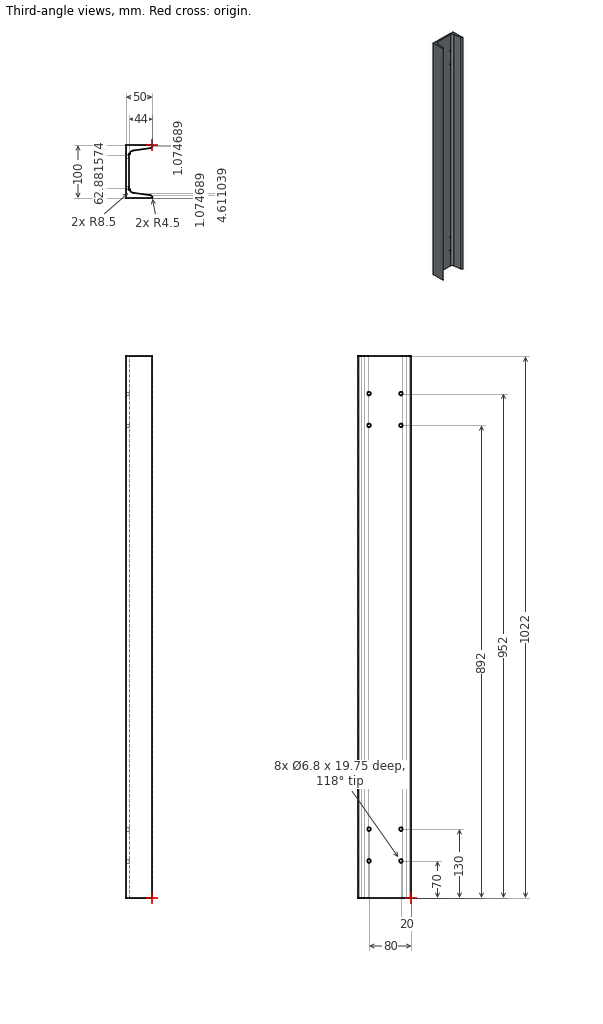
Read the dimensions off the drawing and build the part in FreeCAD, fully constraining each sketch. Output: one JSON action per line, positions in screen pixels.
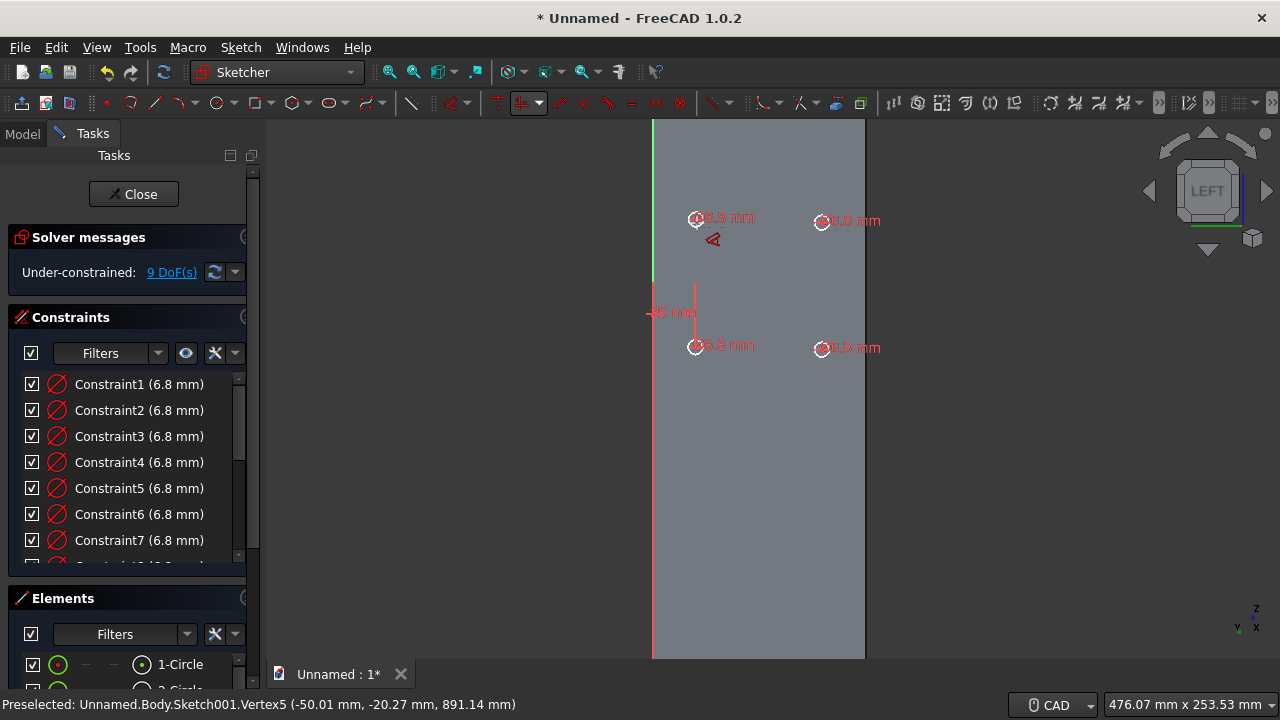
{"action": "left_click", "coordinate": [696, 220]}
{"action": "left_click", "coordinate": [674, 186]}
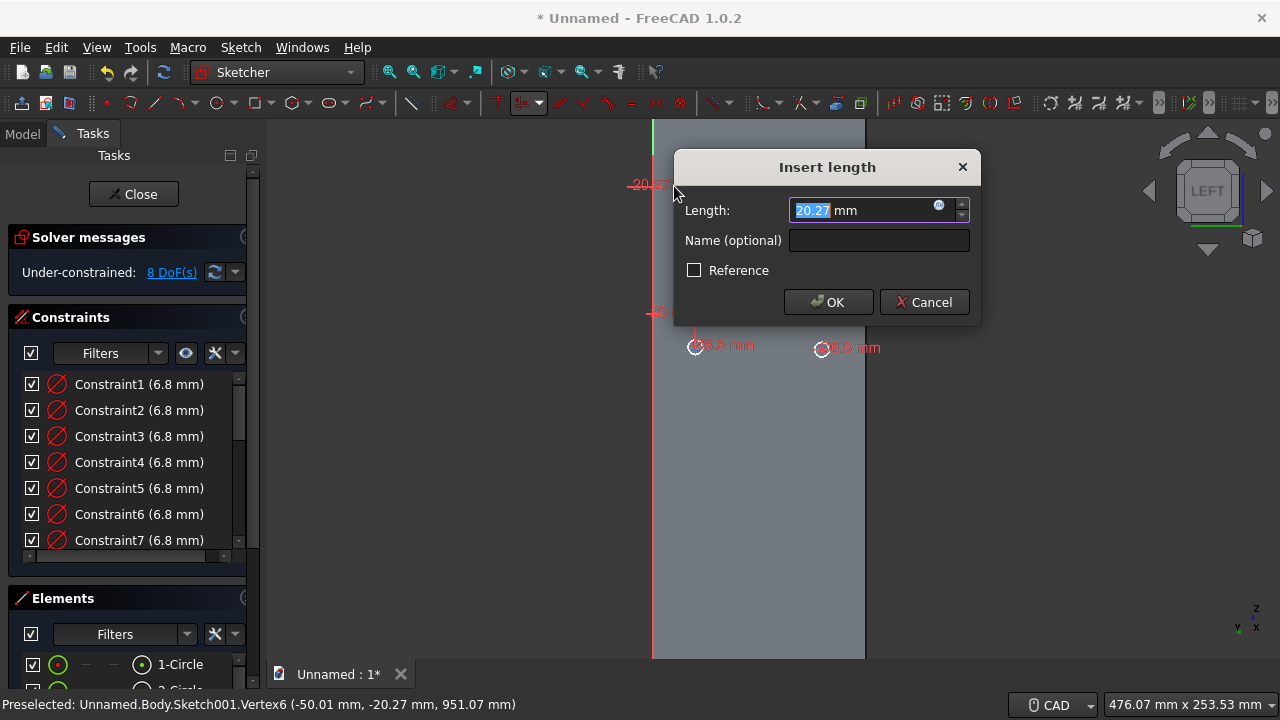
{"action": "type", "text": "20"}
{"action": "key", "text": "Return"}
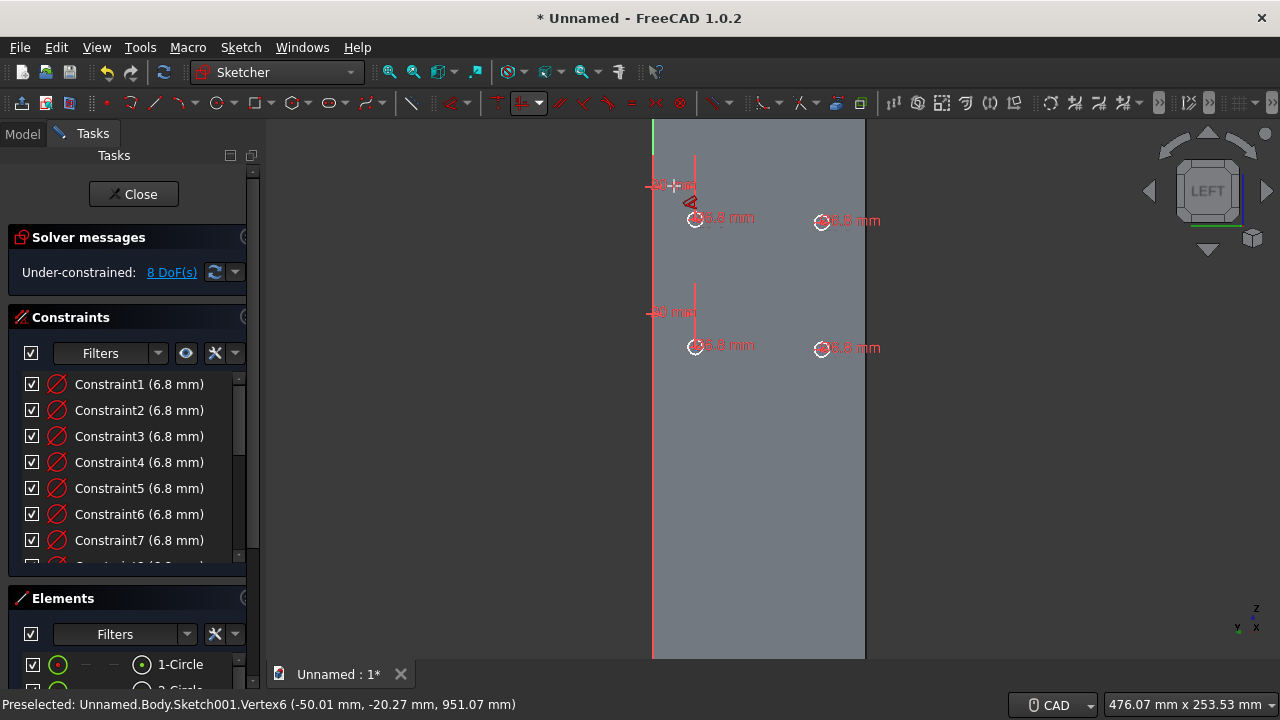
{"action": "scroll", "coordinate": [697, 223], "scroll_direction": "down", "scroll_amount": 9}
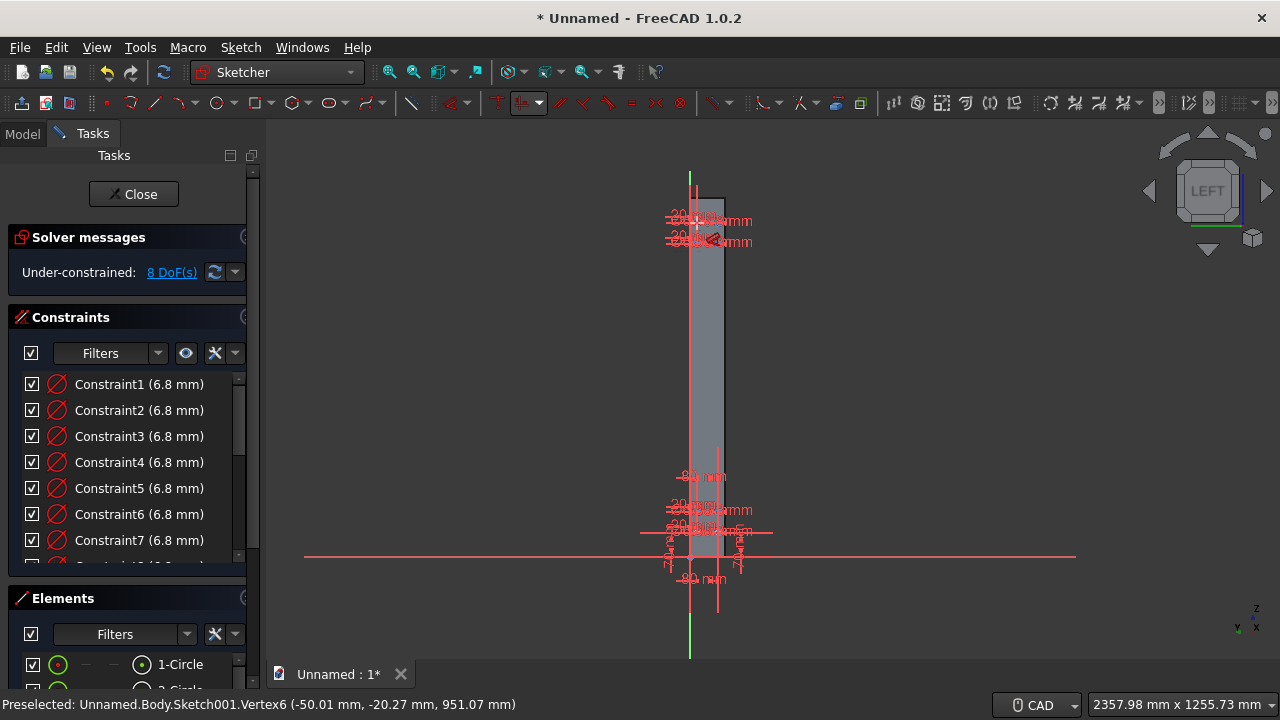
{"action": "scroll", "coordinate": [718, 223], "scroll_direction": "up", "scroll_amount": 2}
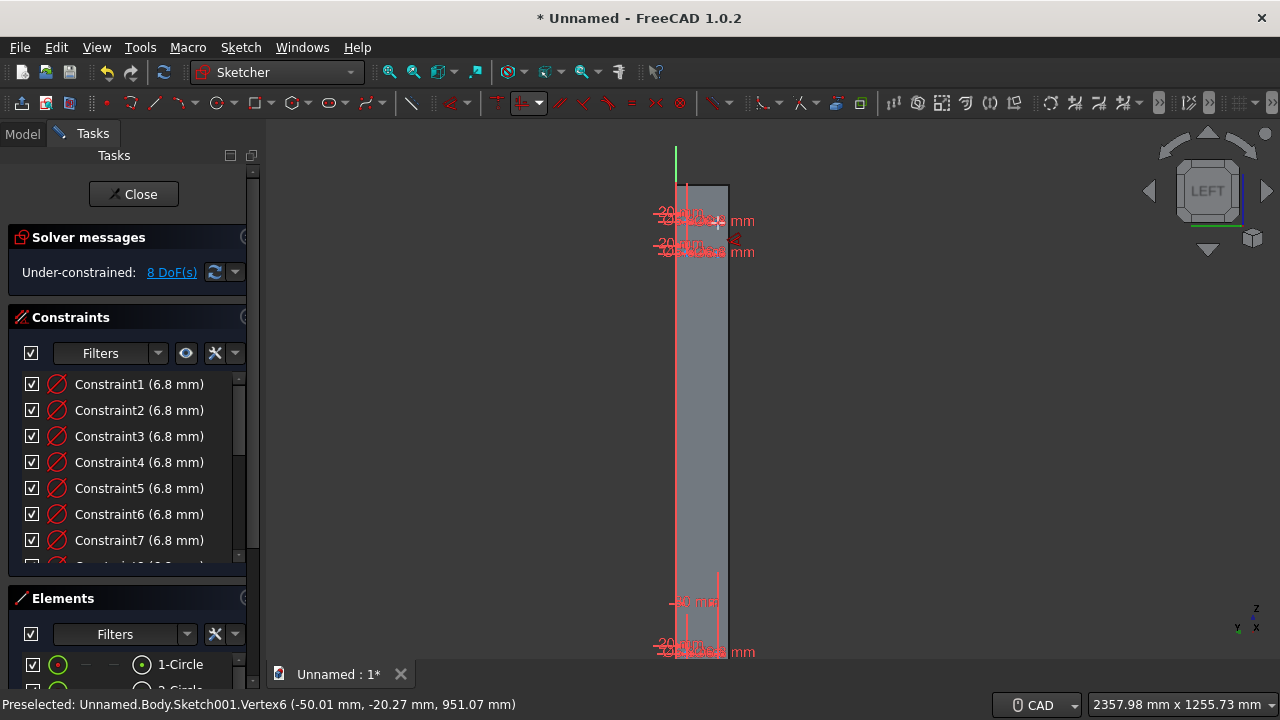
{"action": "left_click", "coordinate": [718, 223]}
{"action": "left_click", "coordinate": [697, 189]}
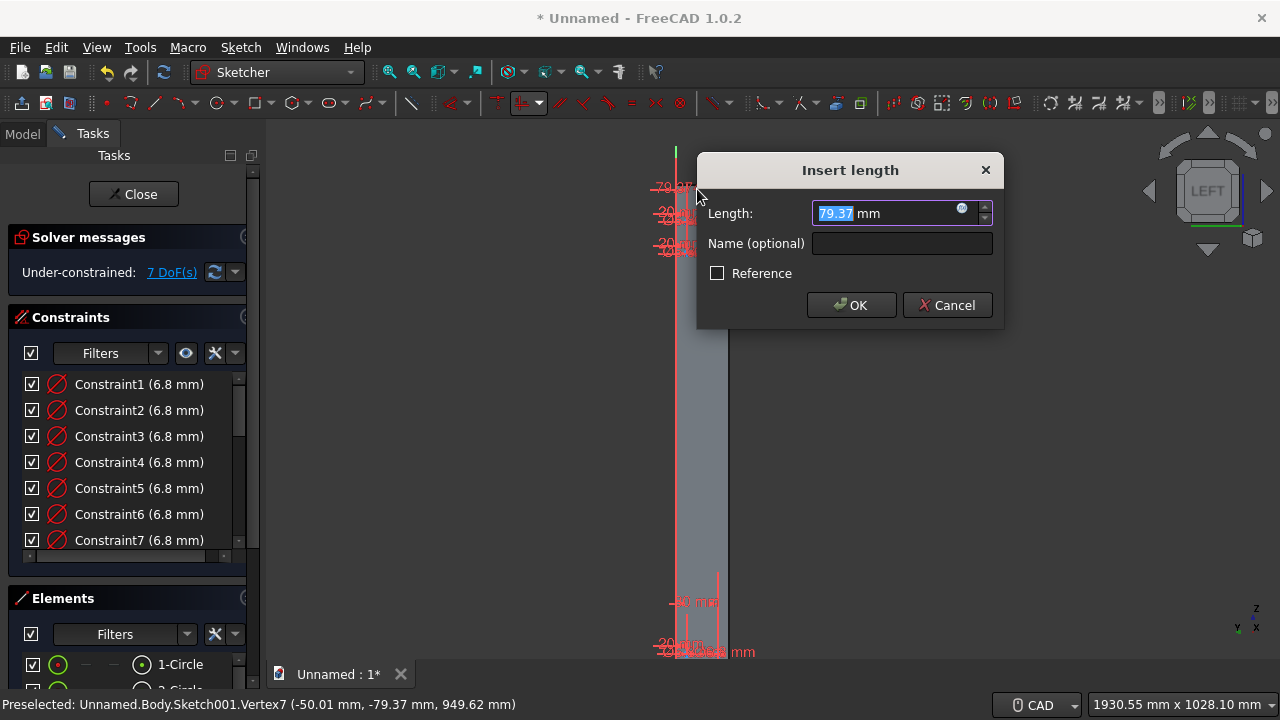
{"action": "type", "text": "80"}
{"action": "key", "text": "Return"}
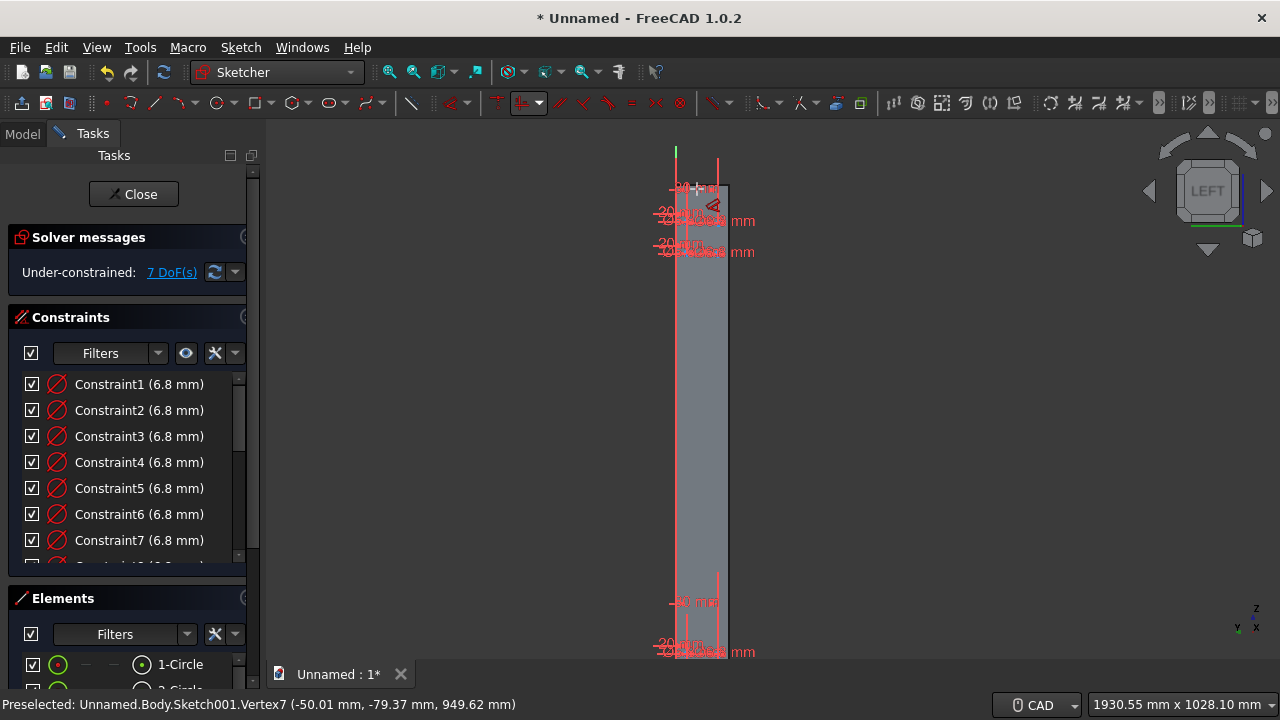
{"action": "left_click", "coordinate": [718, 254]}
{"action": "left_click", "coordinate": [697, 148]}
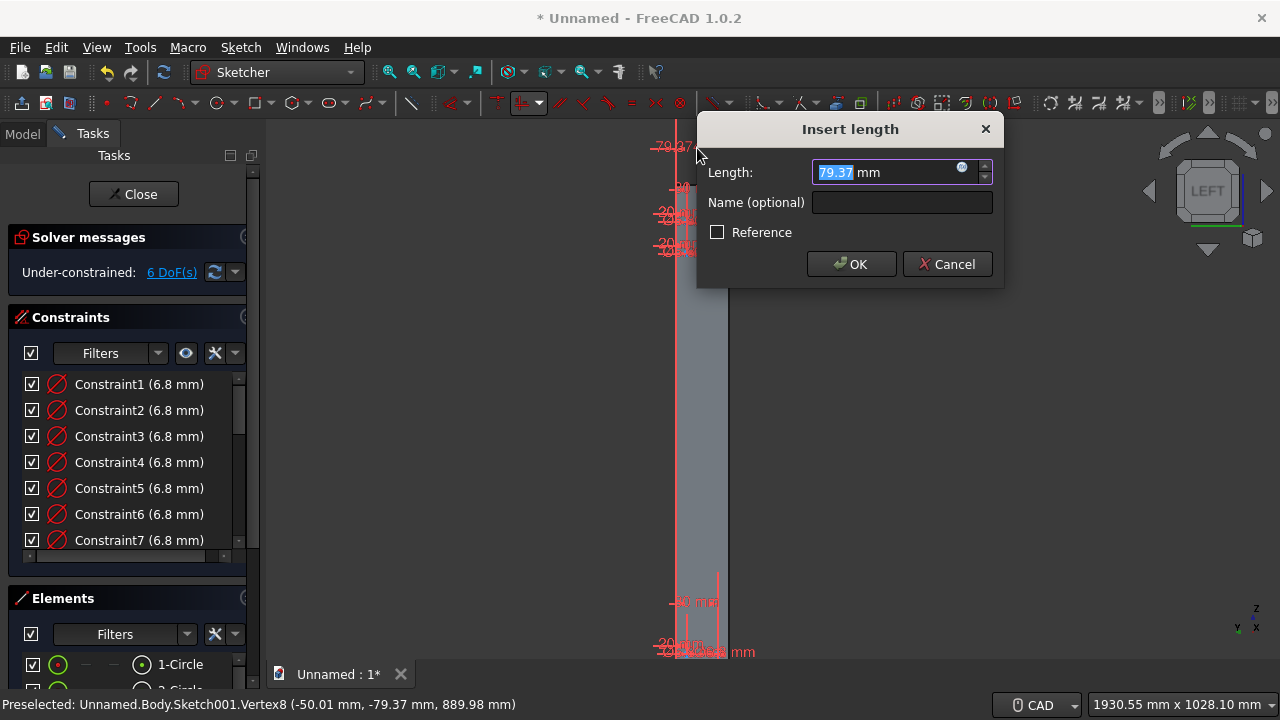
{"action": "type", "text": "80"}
{"action": "key", "text": "Return"}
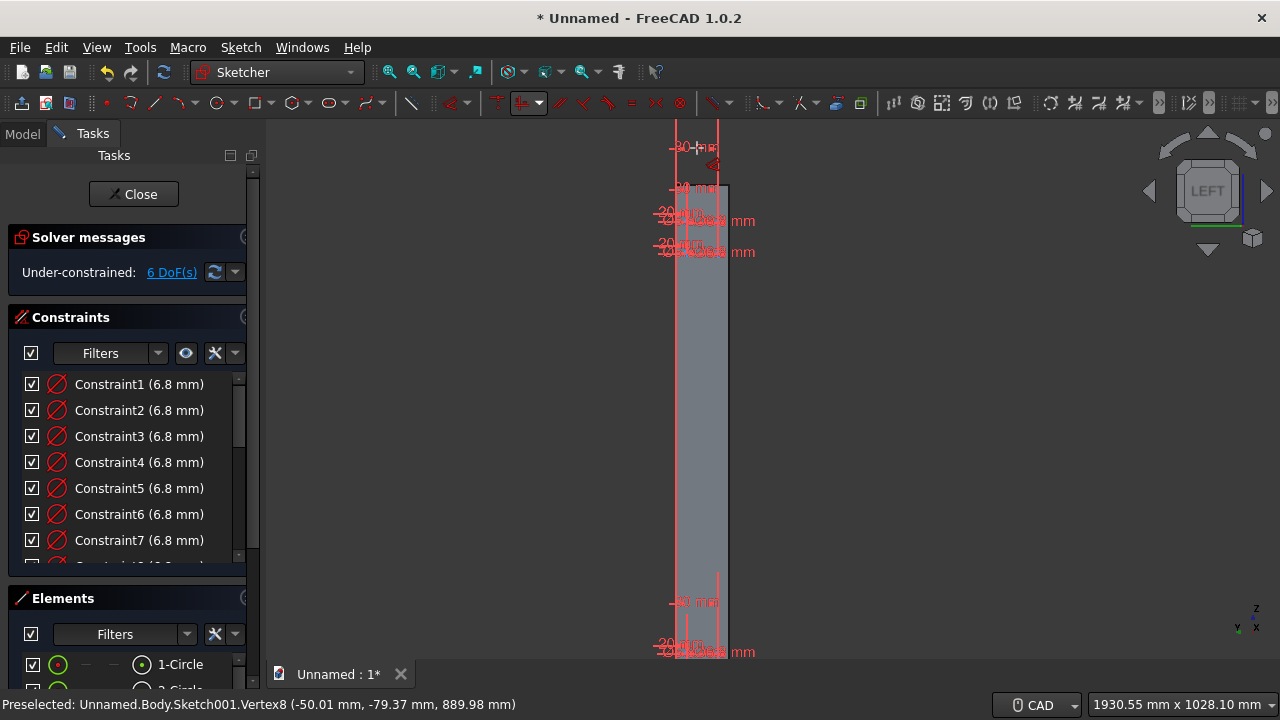
{"action": "scroll", "coordinate": [718, 222], "scroll_direction": "down", "scroll_amount": 2}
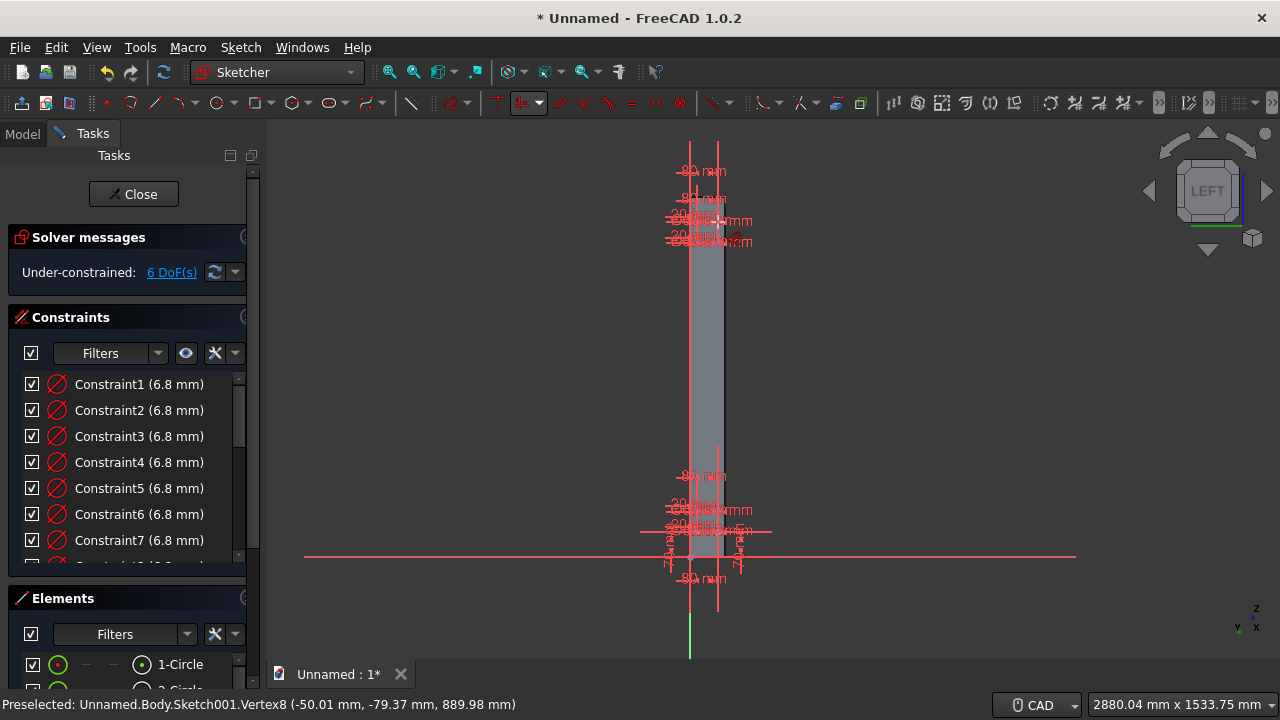
{"action": "left_click", "coordinate": [697, 512]}
{"action": "left_click", "coordinate": [608, 524]}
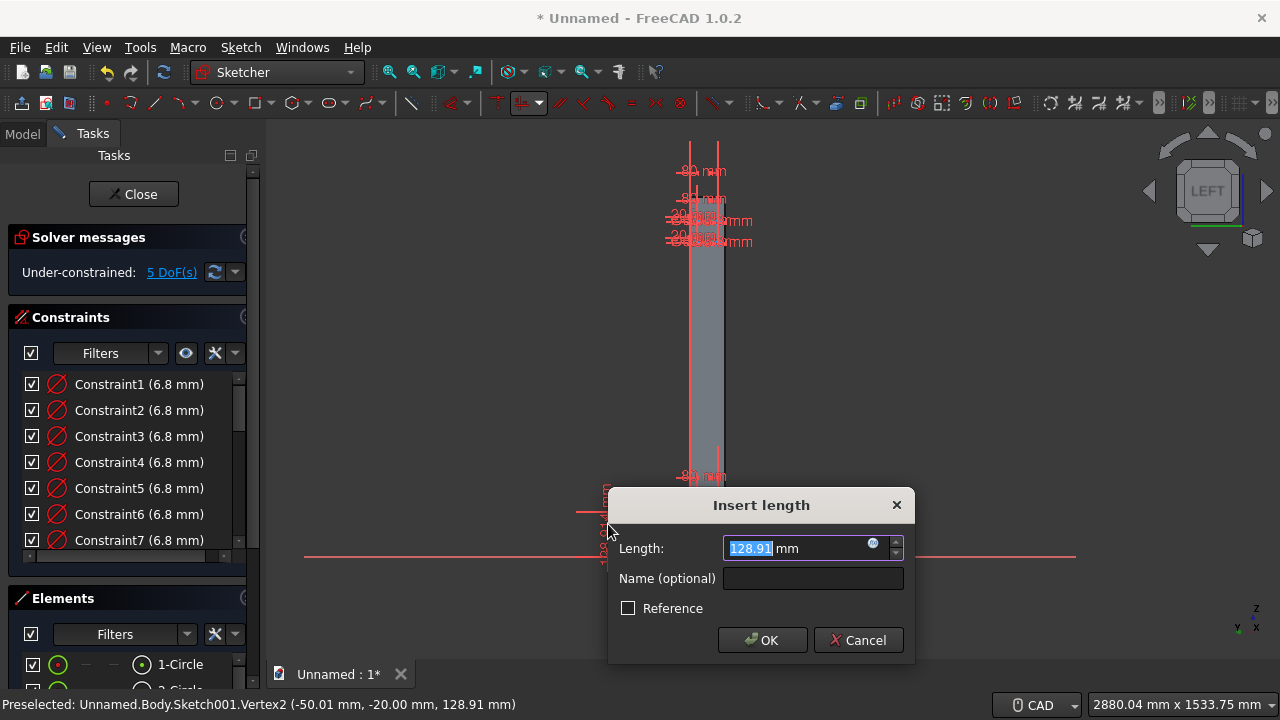
{"action": "type", "text": "130"}
{"action": "key", "text": "Return"}